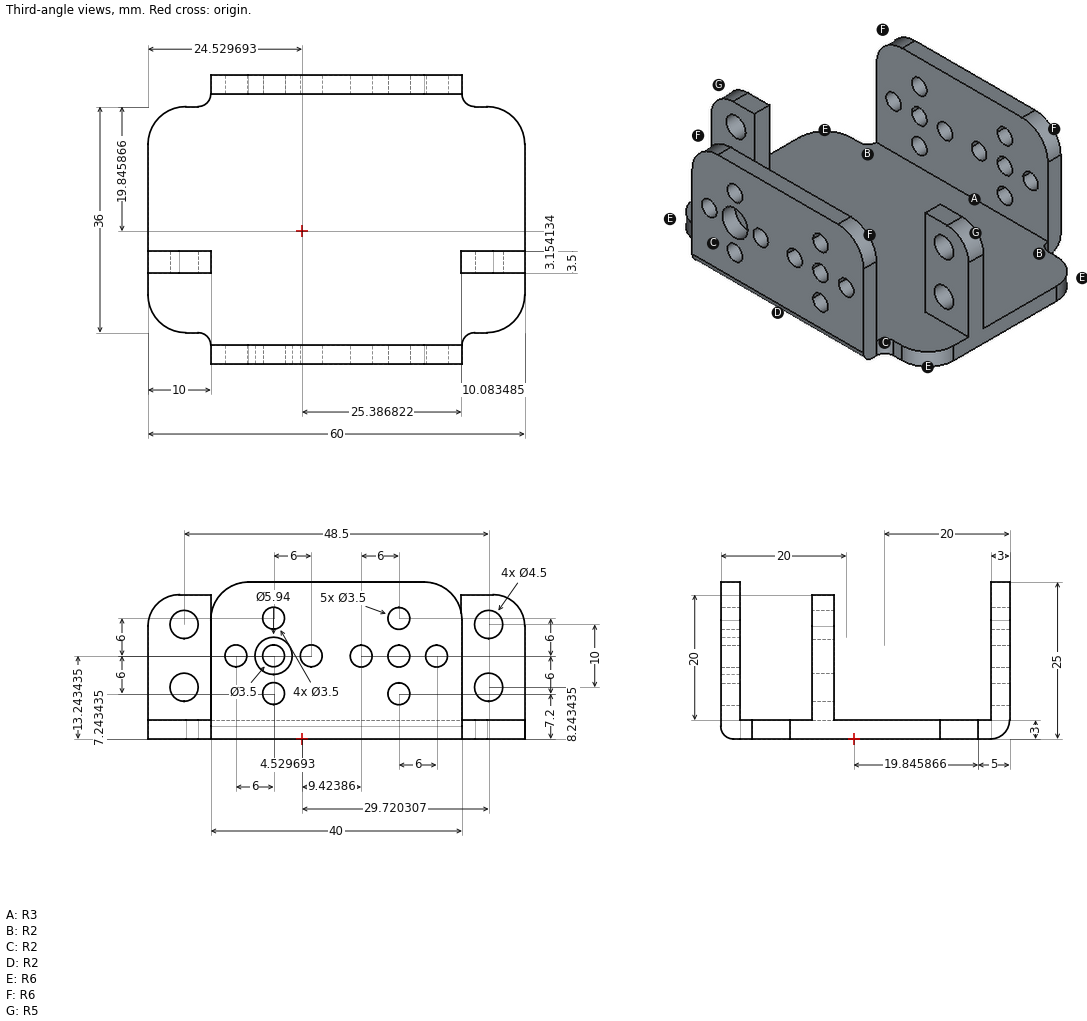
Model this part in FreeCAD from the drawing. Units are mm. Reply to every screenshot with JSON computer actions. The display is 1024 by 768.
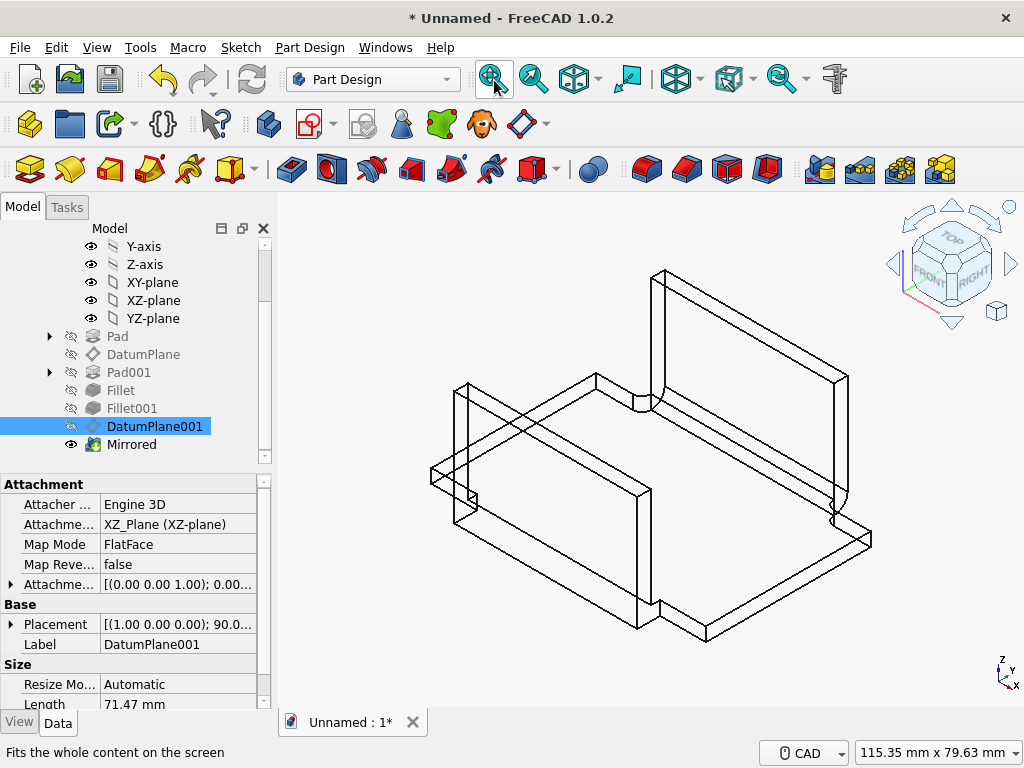
{"action": "left_click", "coordinate": [660, 607]}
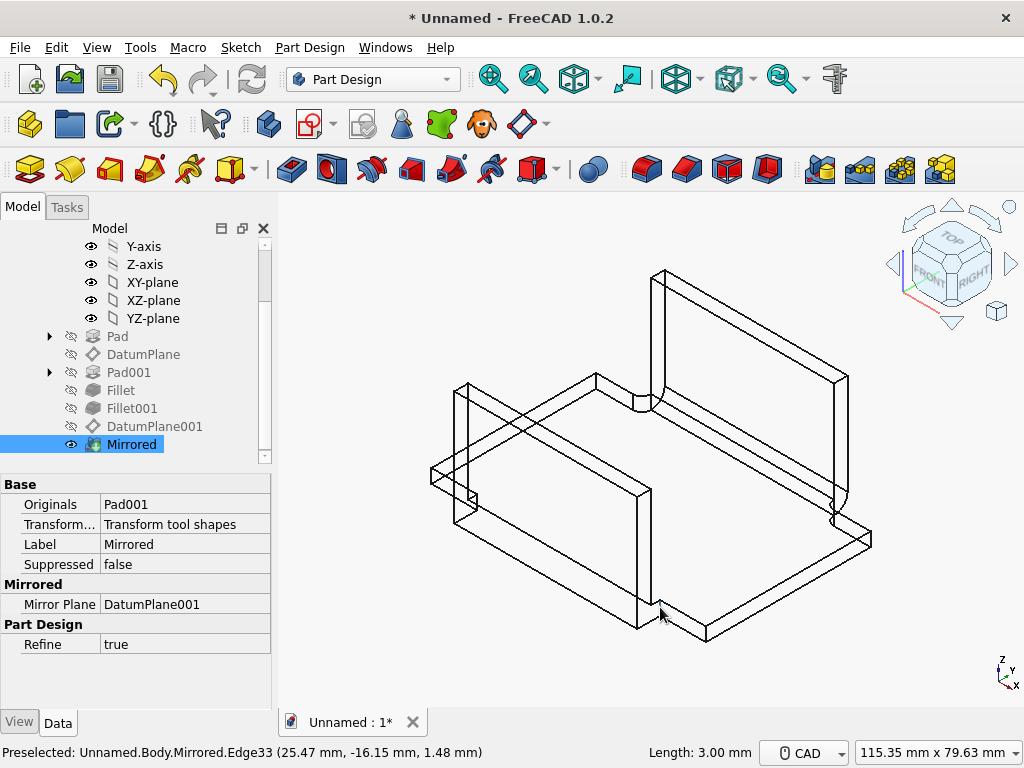
{"action": "scroll", "coordinate": [477, 501], "scroll_direction": "up", "scroll_amount": 6}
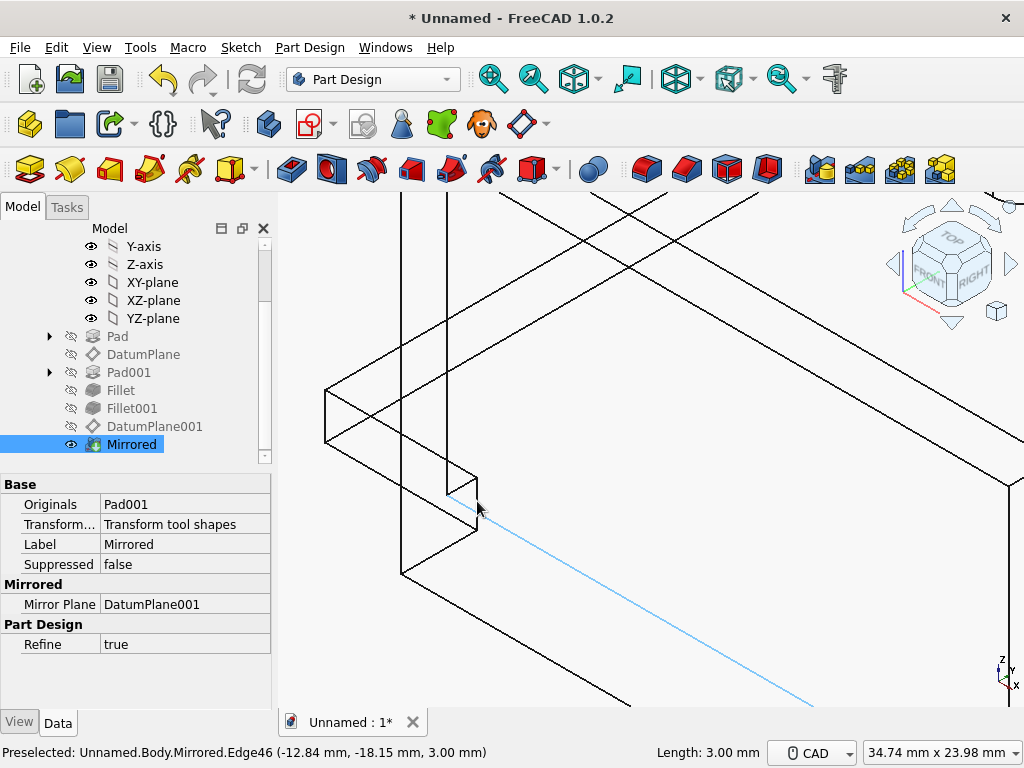
{"action": "left_click", "coordinate": [477, 503], "text": "ctrl"}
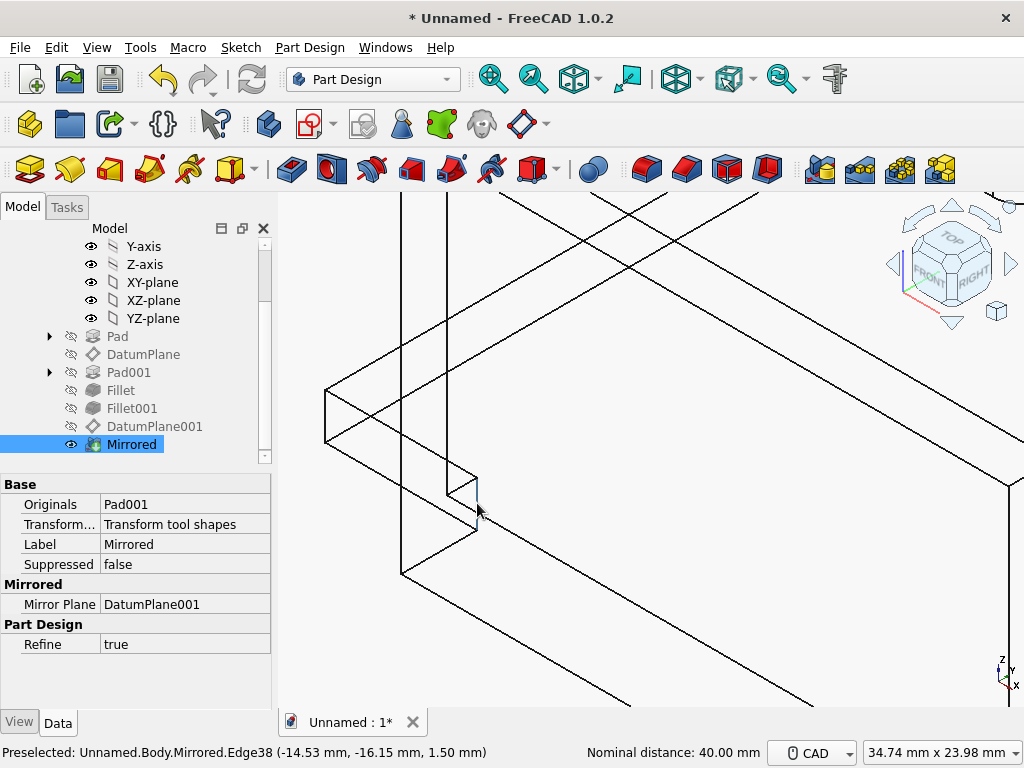
{"action": "key", "text": "v 1"}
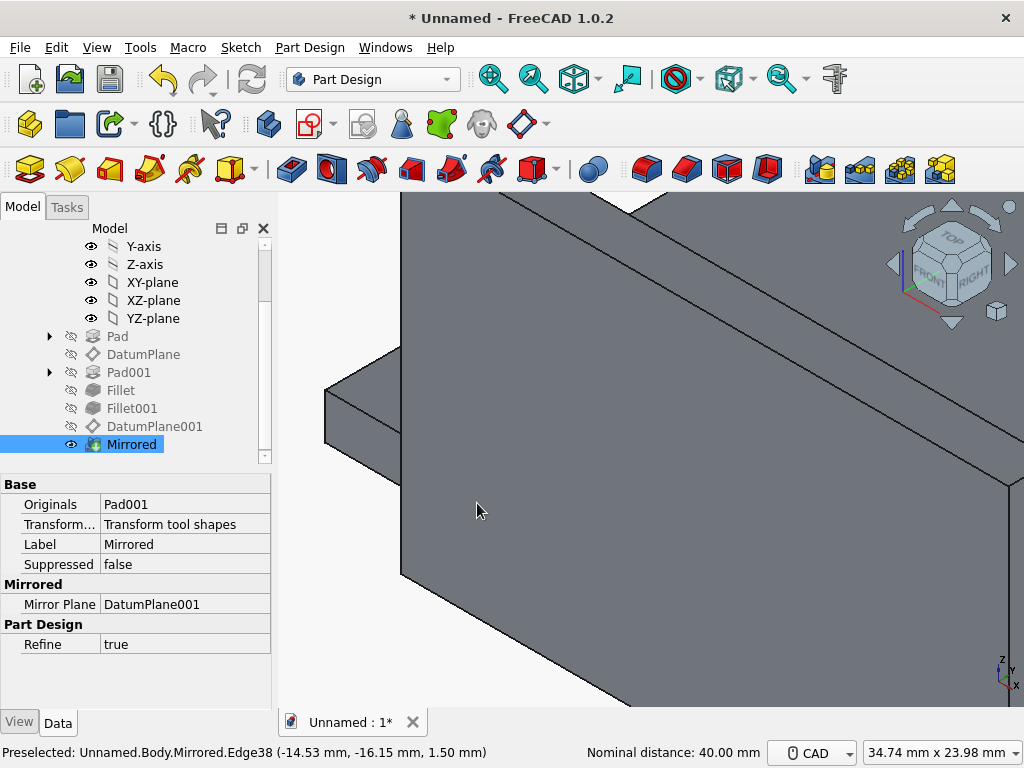
{"action": "left_click", "coordinate": [648, 170]}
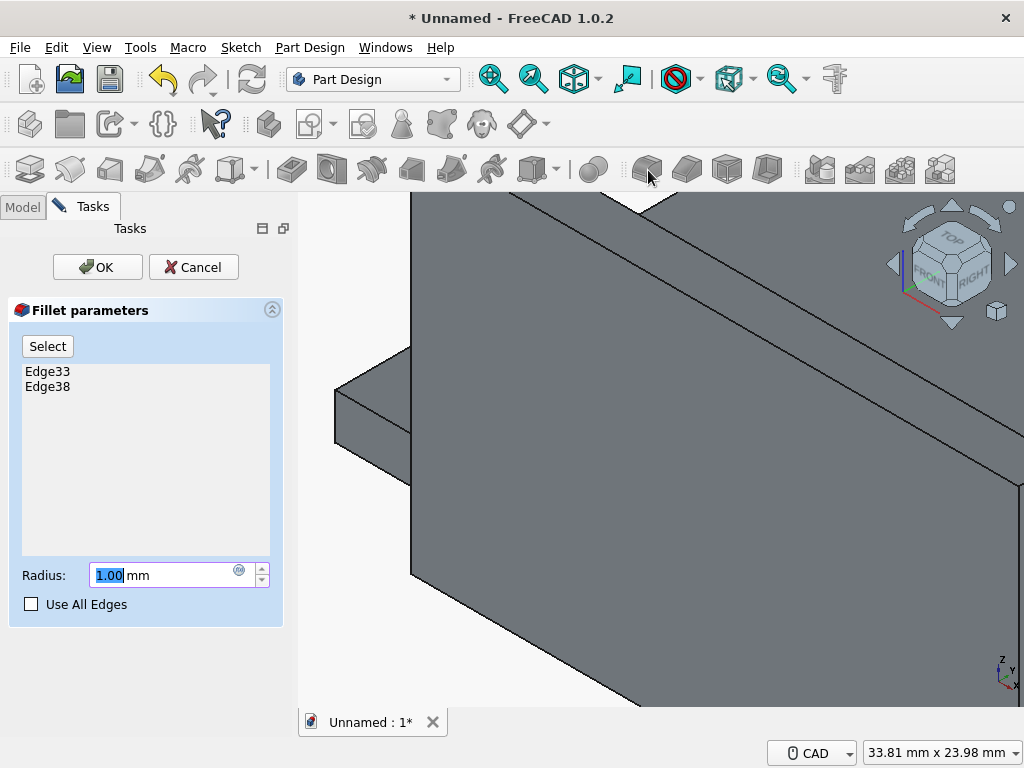
{"action": "type", "text": "2"}
{"action": "key", "text": "Tab"}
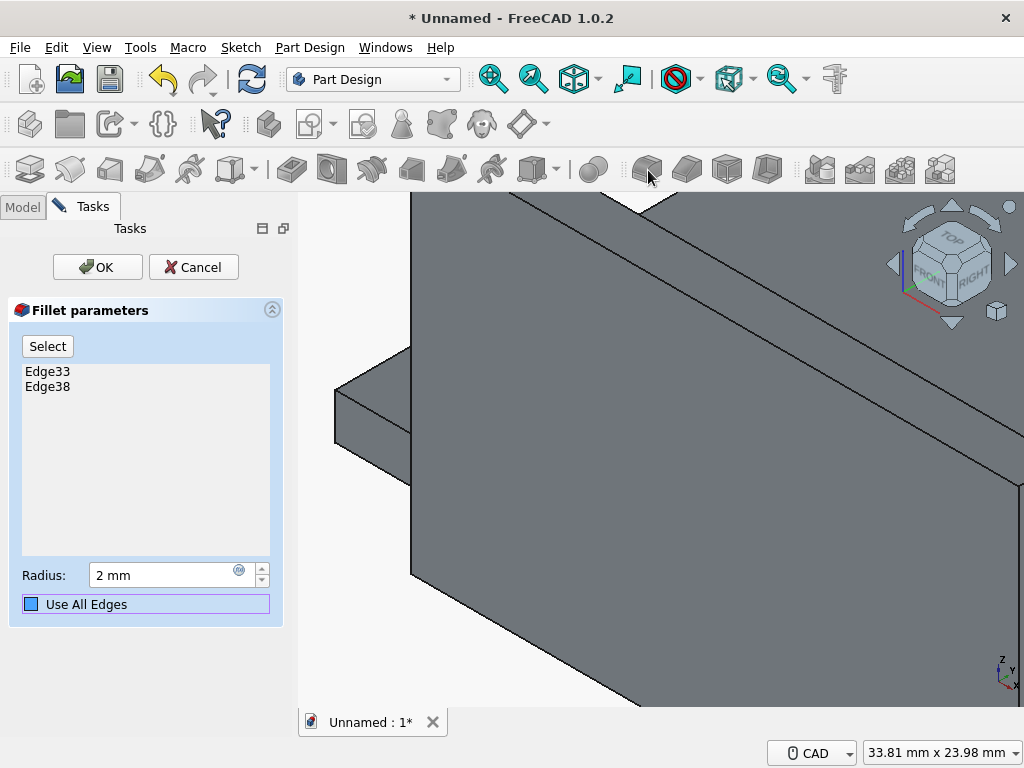
{"action": "left_click", "coordinate": [98, 267]}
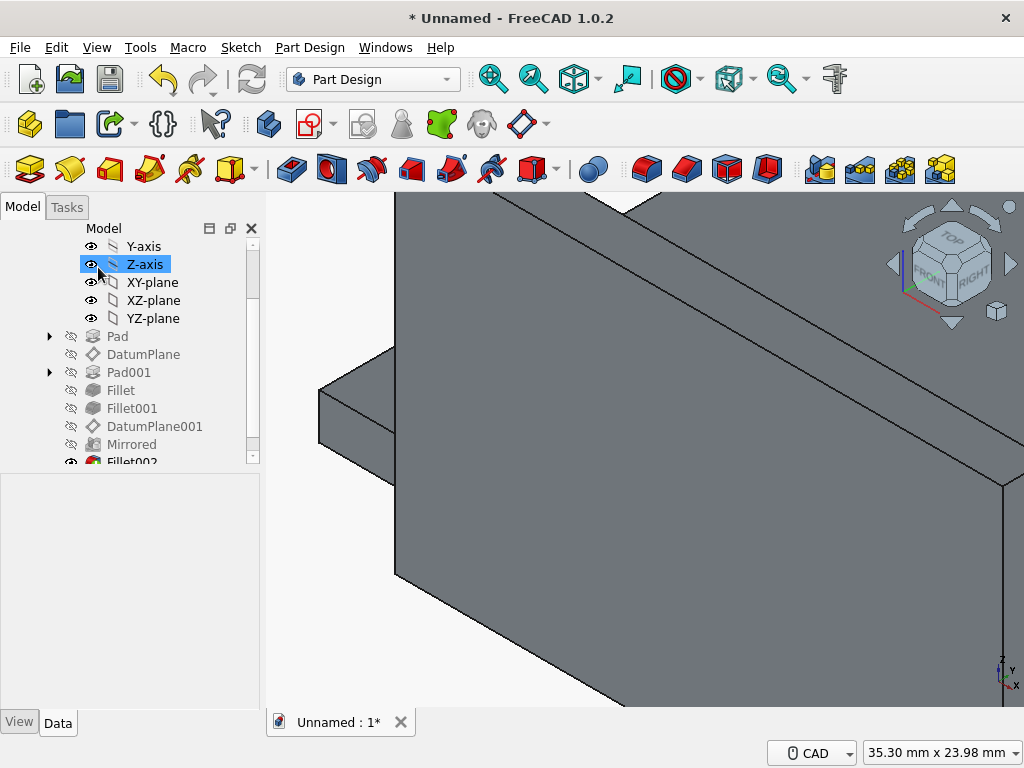
{"action": "left_click", "coordinate": [494, 80]}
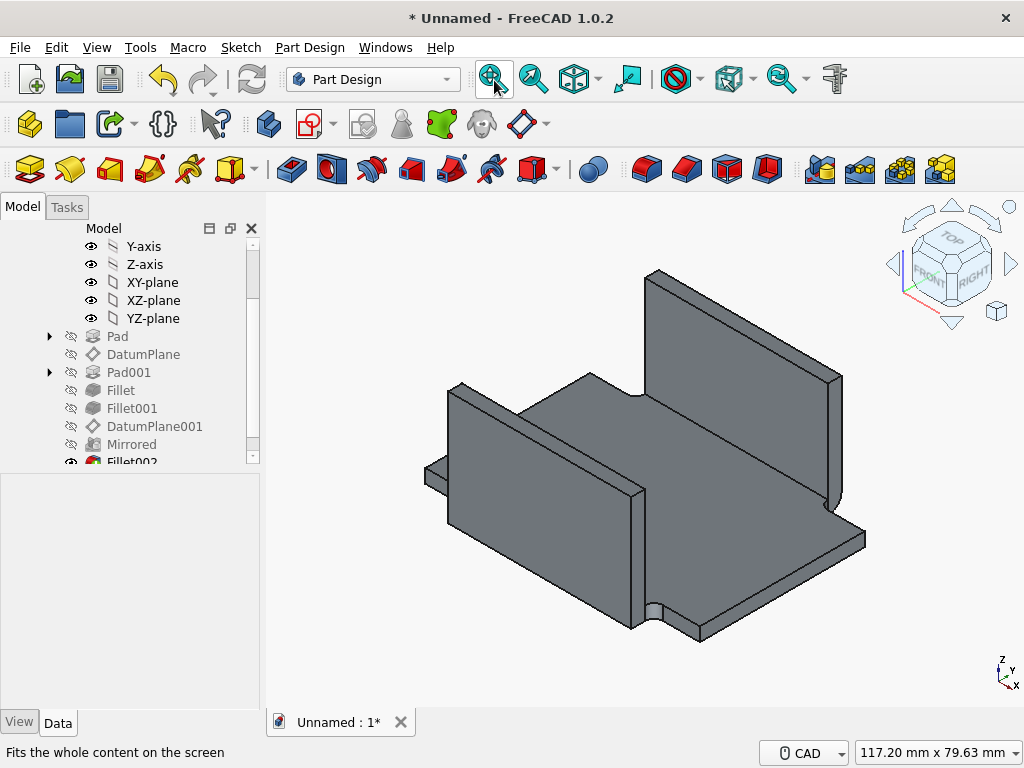
{"action": "key", "text": "2"}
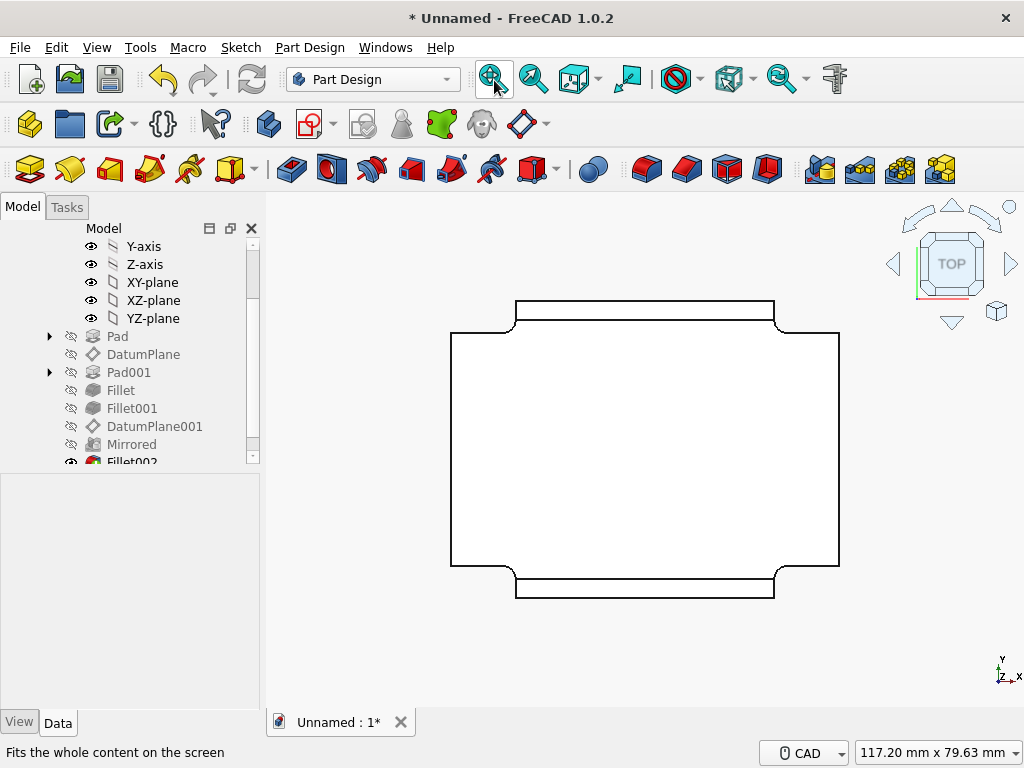
{"action": "key", "text": "0"}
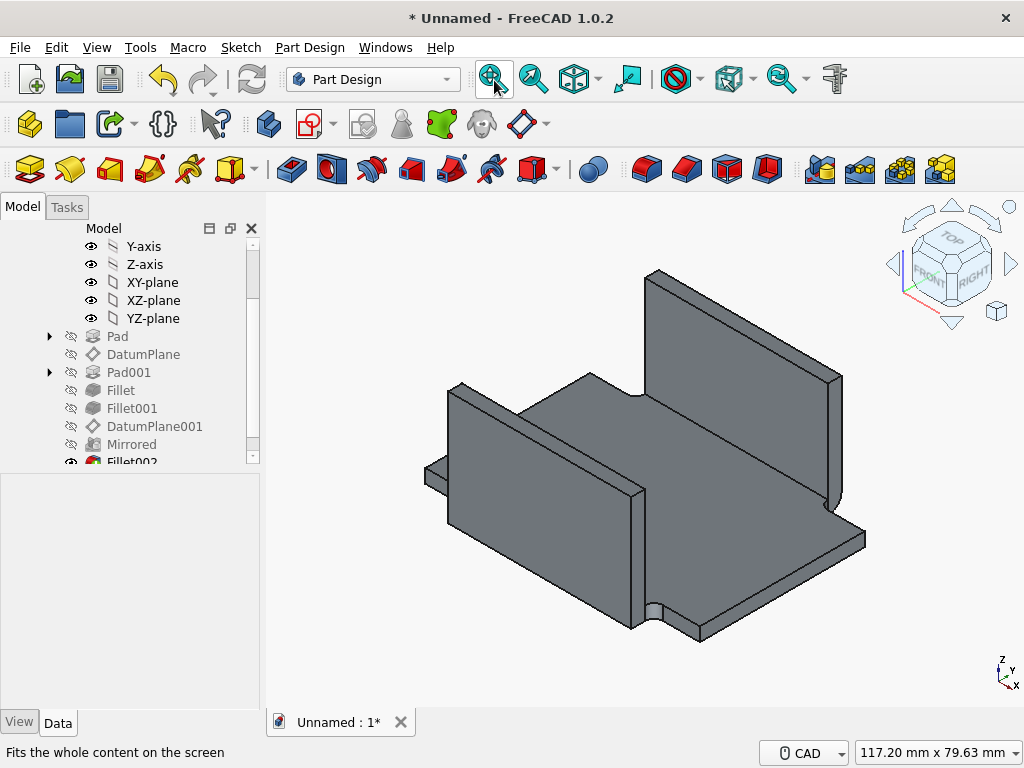
{"action": "key", "text": "1"}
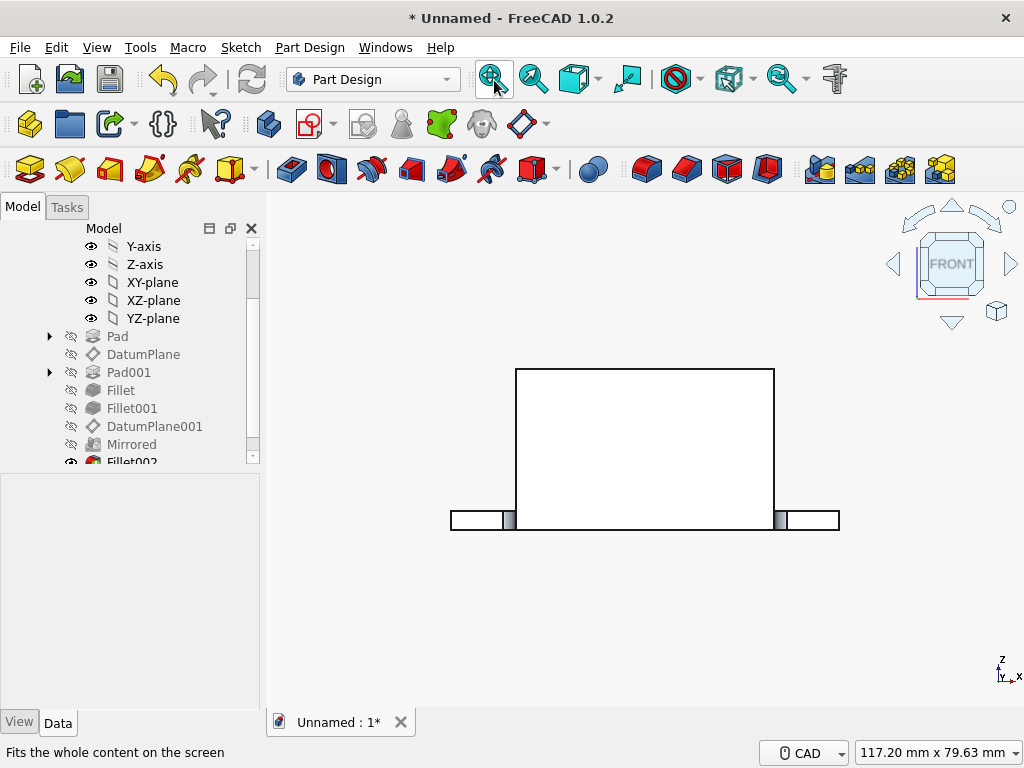
{"action": "left_click", "coordinate": [645, 529]}